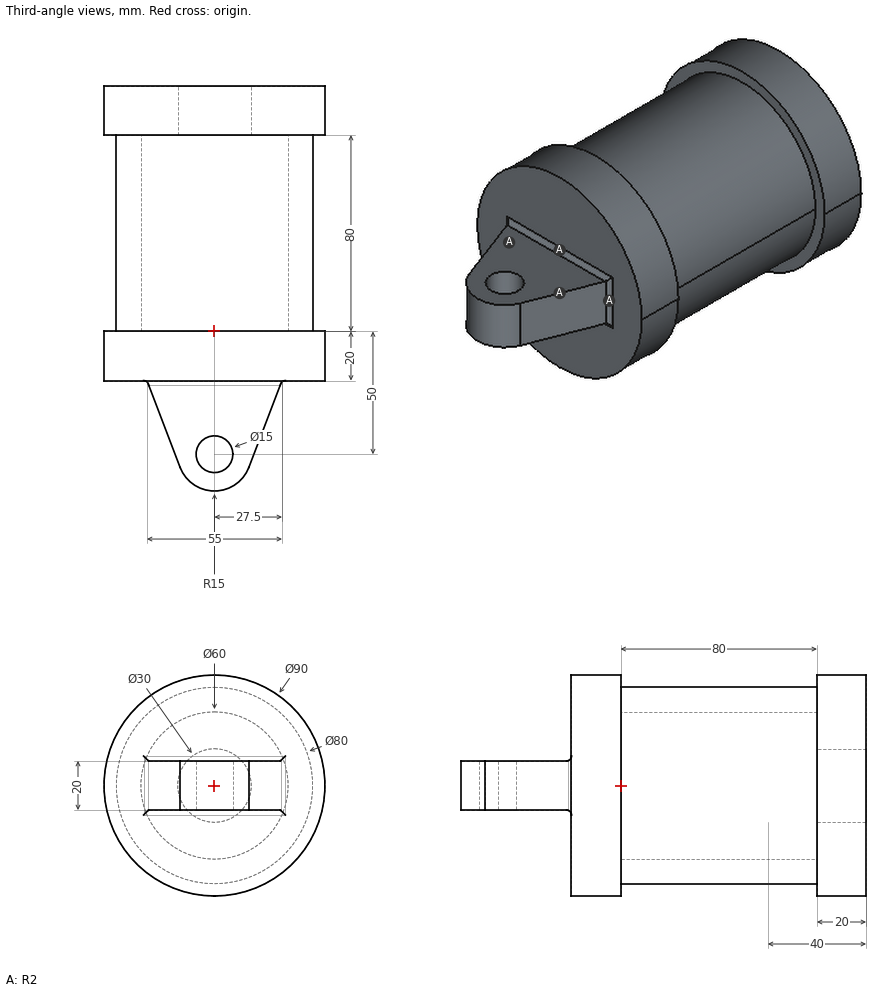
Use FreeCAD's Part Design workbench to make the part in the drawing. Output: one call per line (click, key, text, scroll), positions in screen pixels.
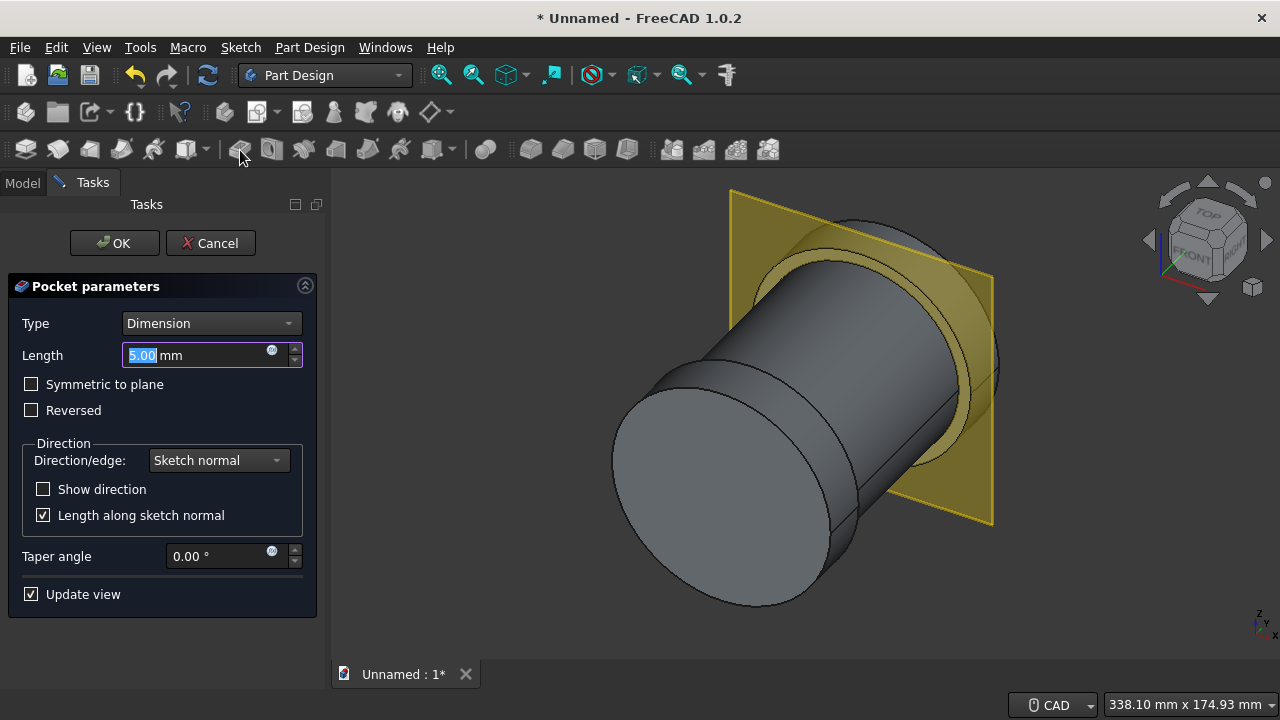
text(80)
key(Tab)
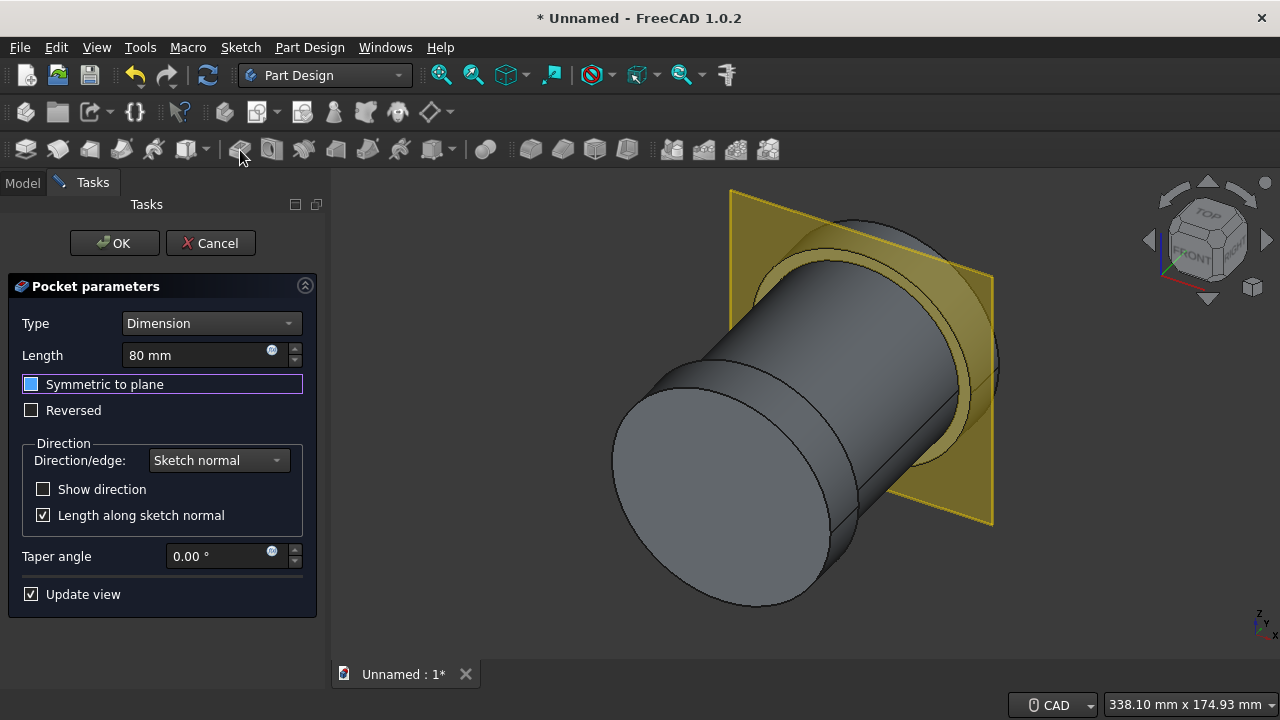
click(30, 410)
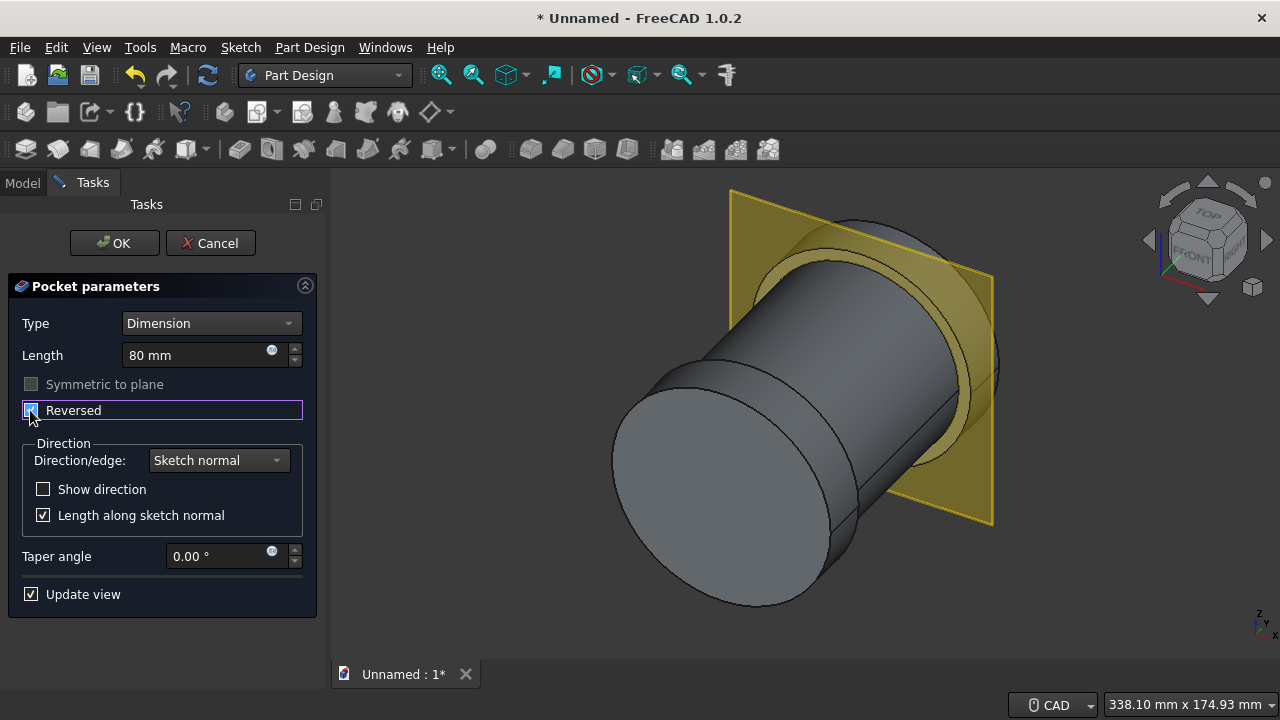
click(115, 243)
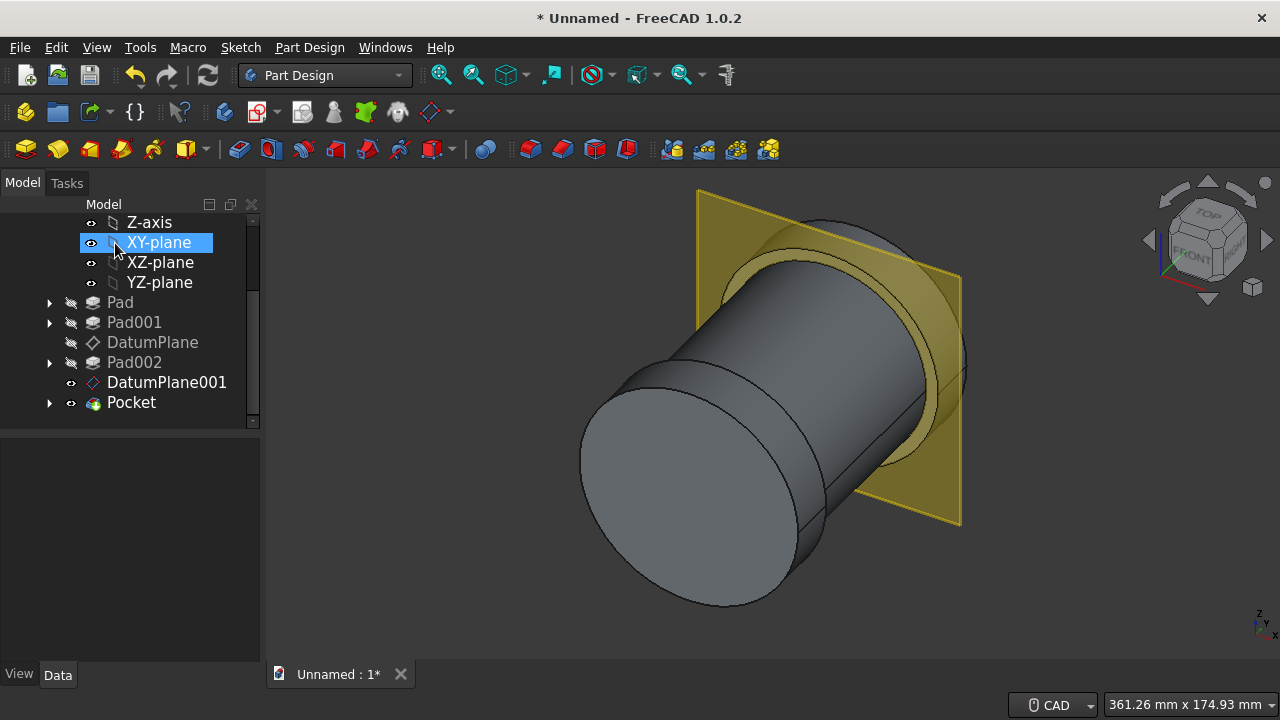
click(116, 383)
key(space)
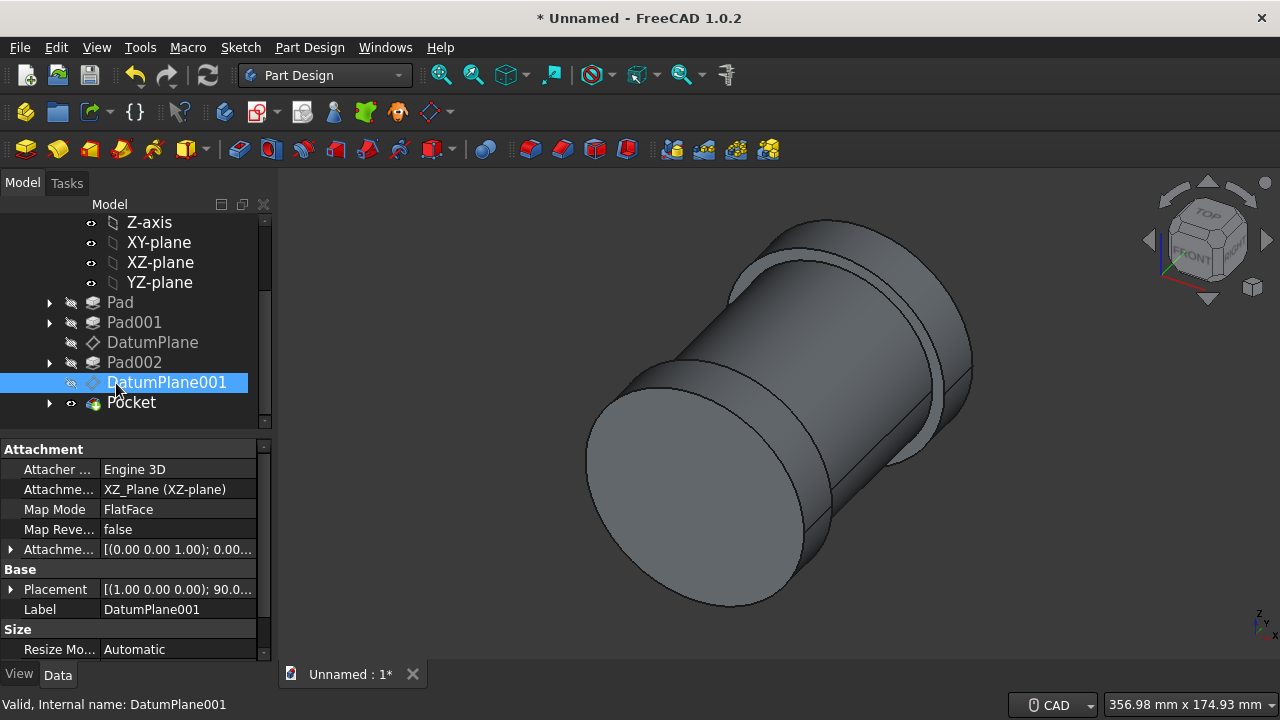
key(4)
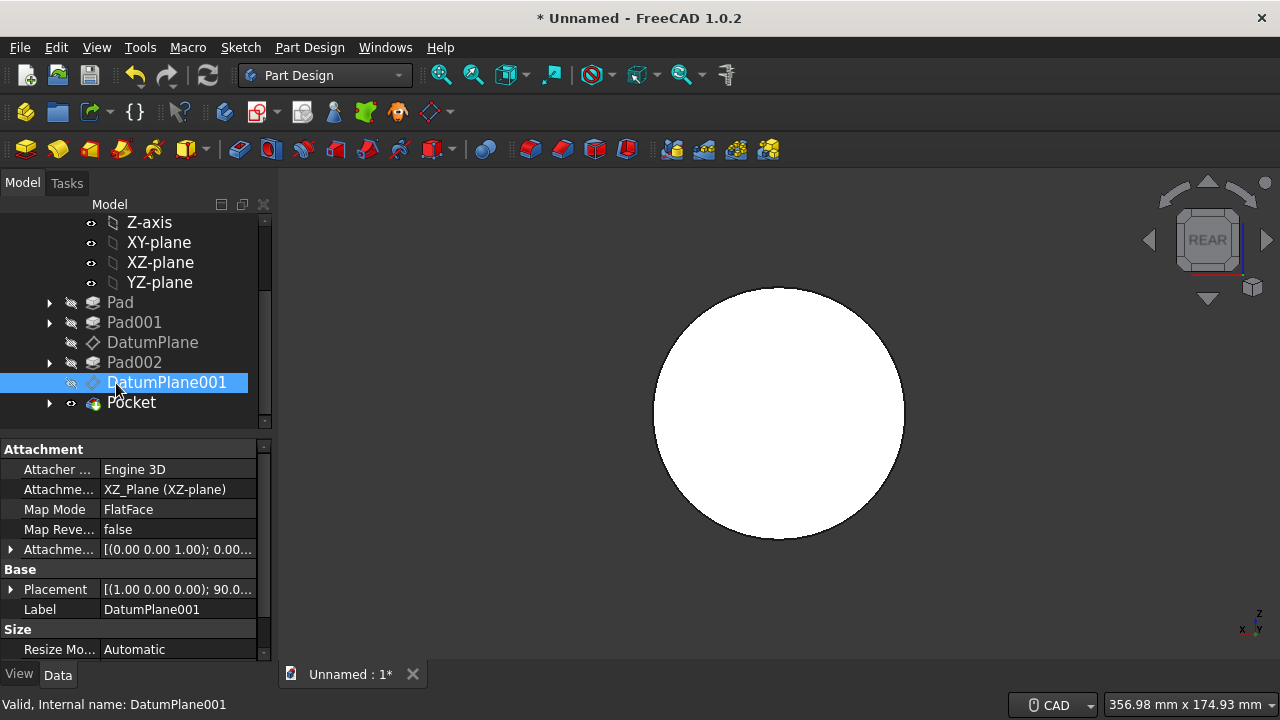
click(779, 412)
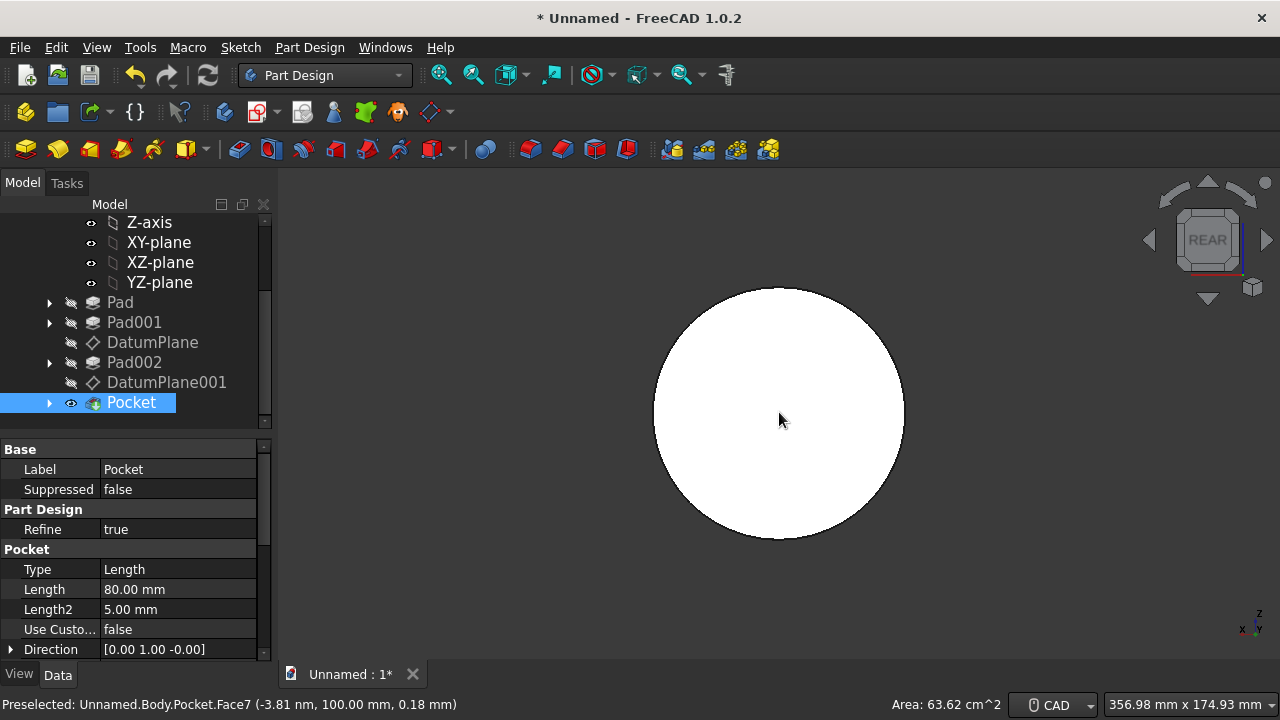
click(258, 112)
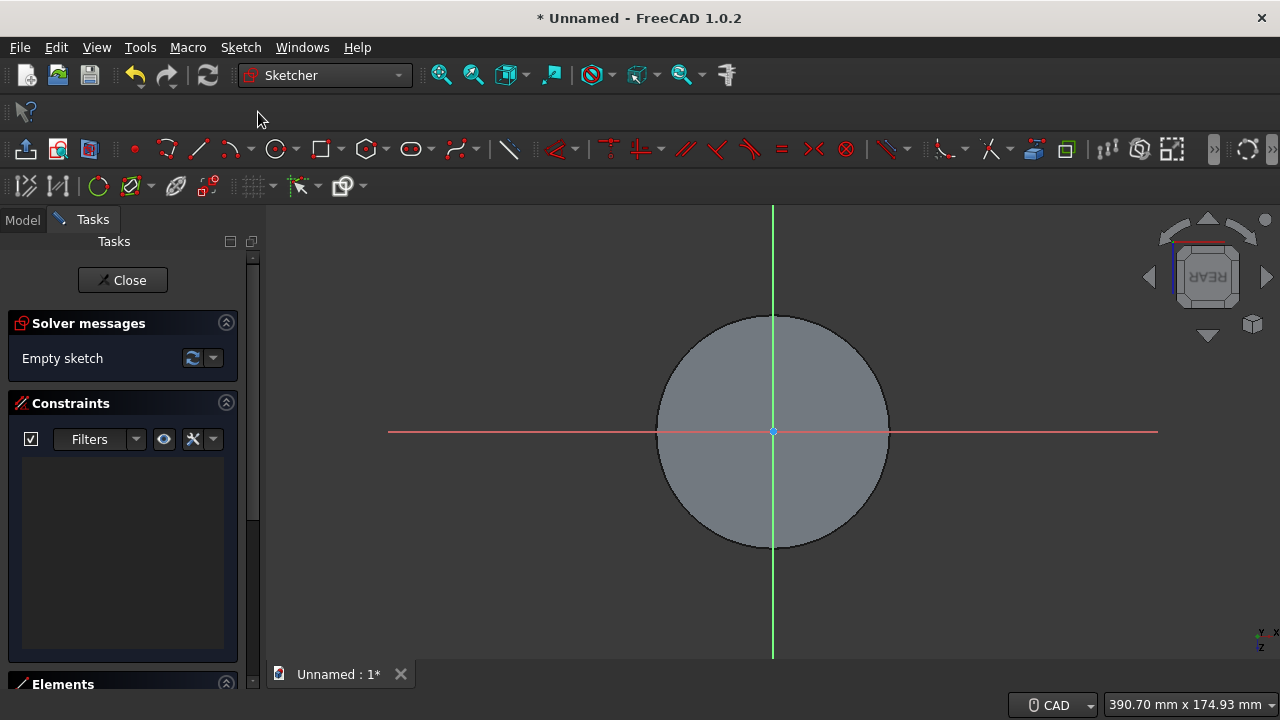
scroll(803, 432, up, 6)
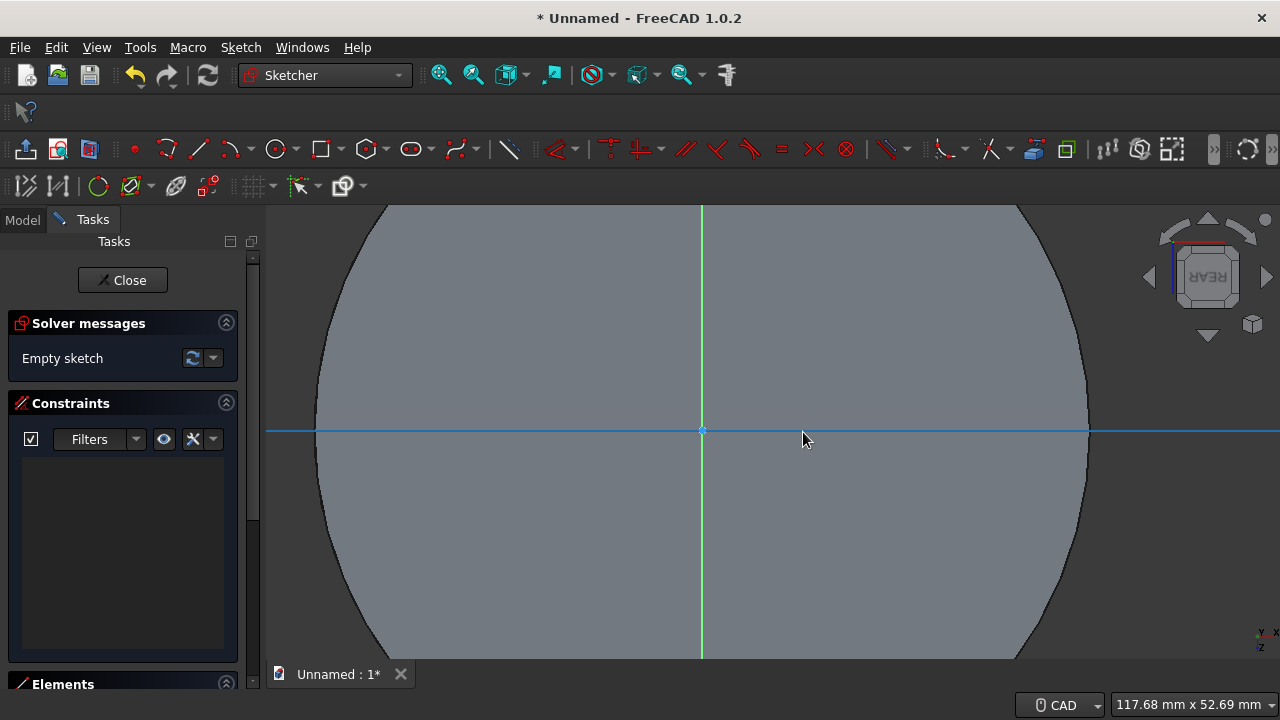
click(276, 150)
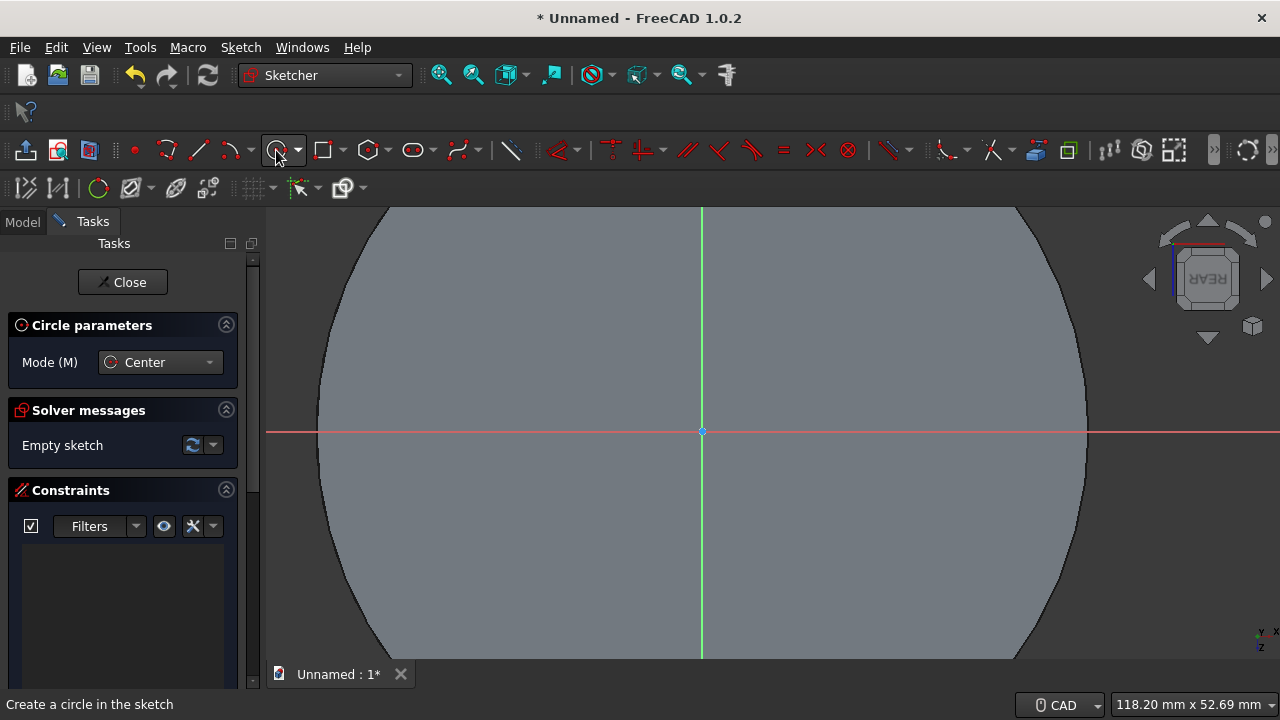
click(702, 432)
move(793, 341)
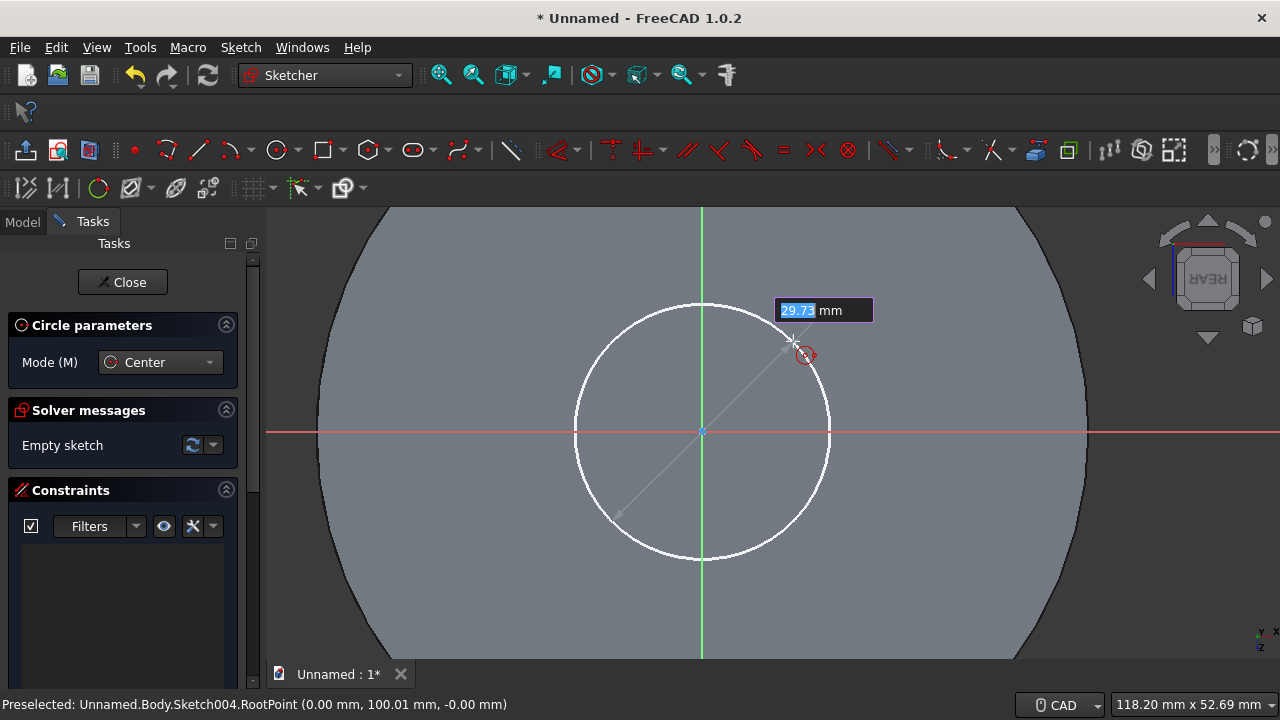
text(30)
key(Return)
key(Escape)